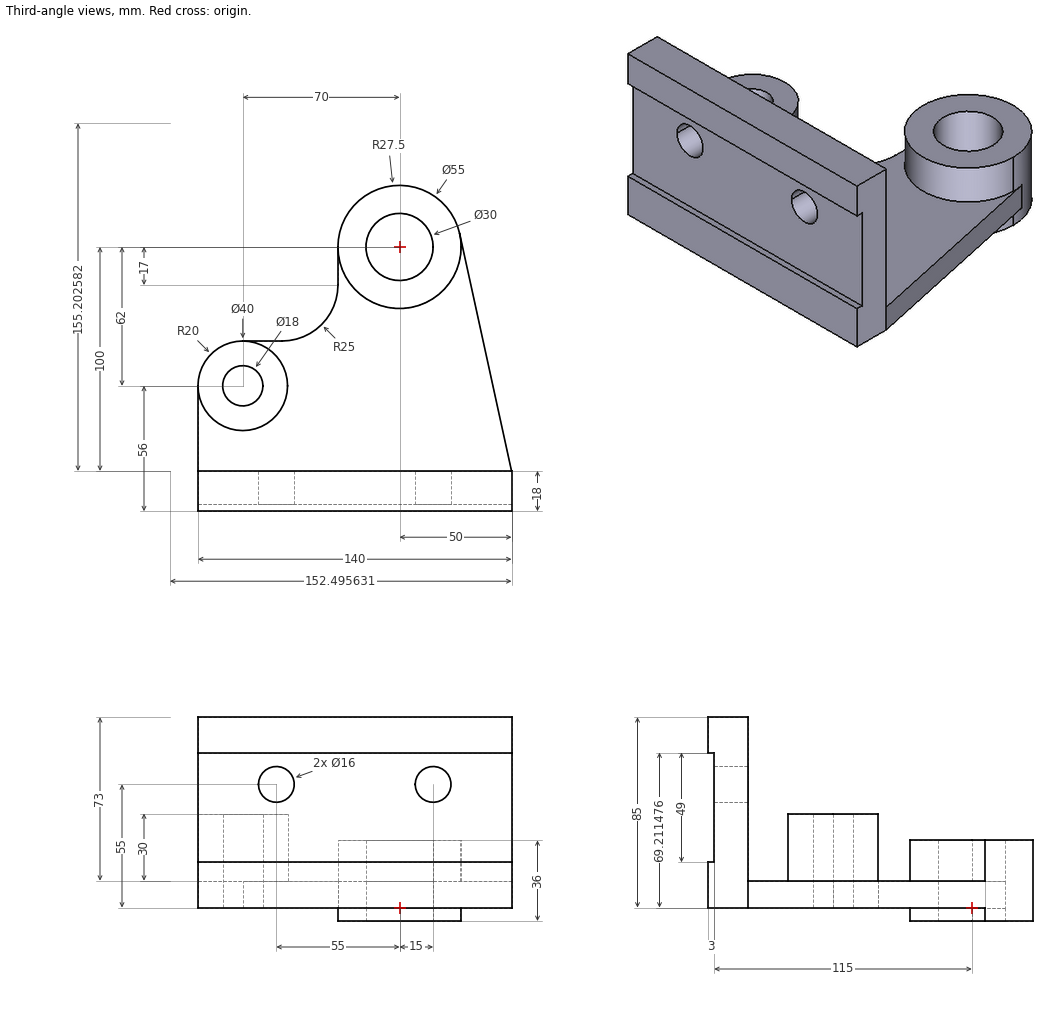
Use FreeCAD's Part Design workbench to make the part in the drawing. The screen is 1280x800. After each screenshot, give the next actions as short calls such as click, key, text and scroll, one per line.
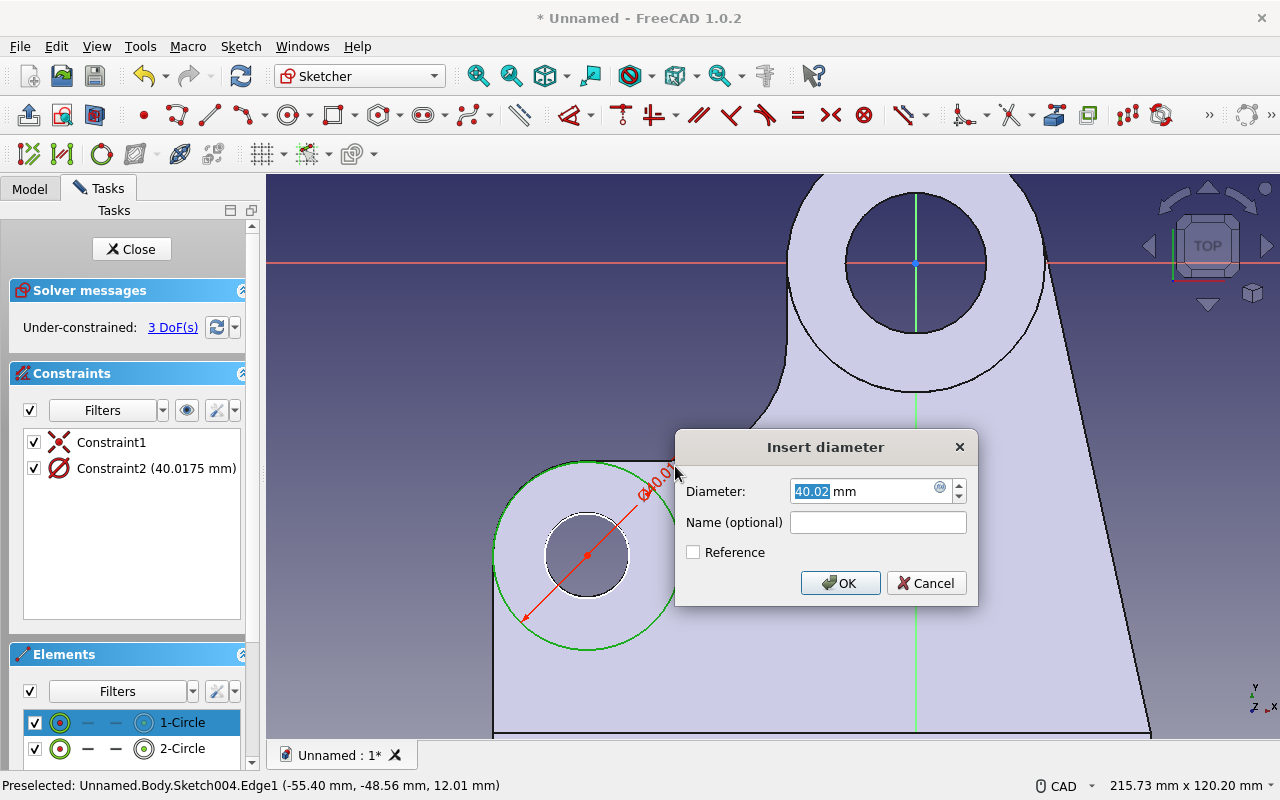
text(40)
key(Return)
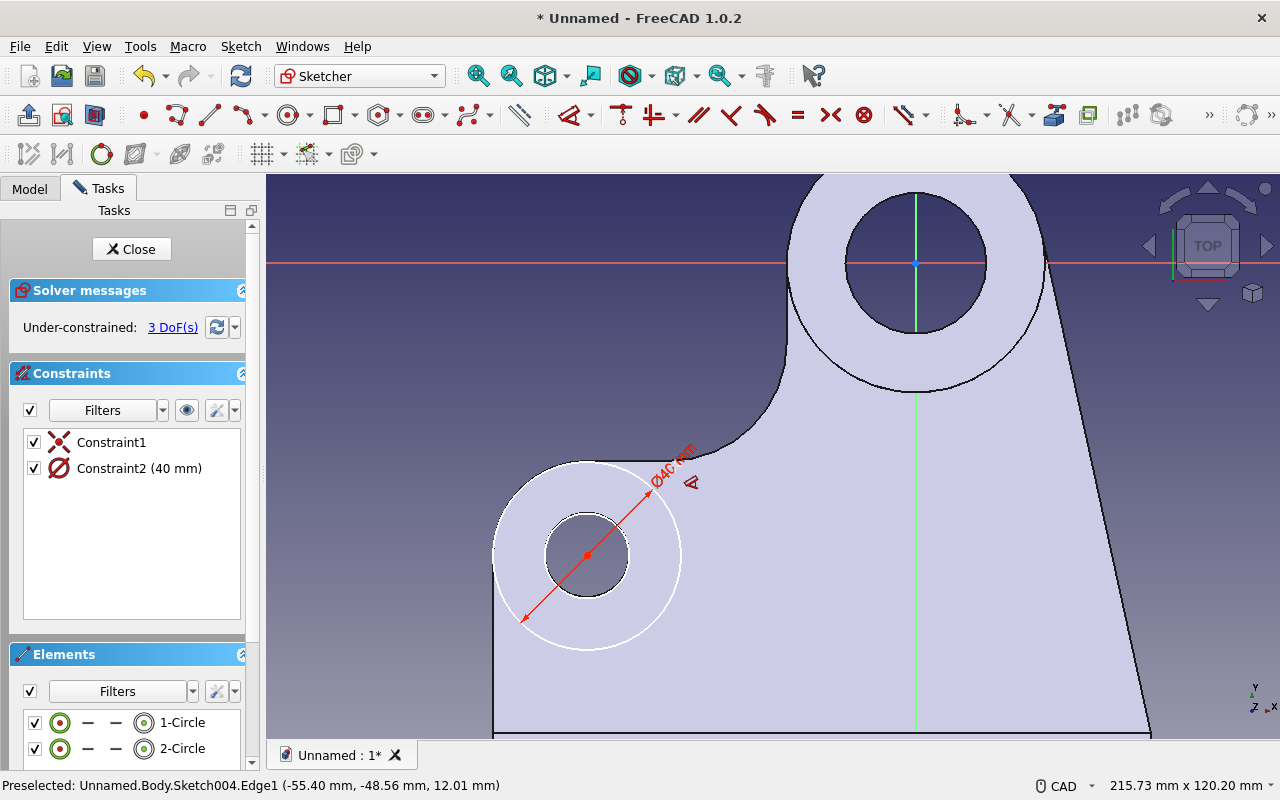
click(617, 526)
click(640, 503)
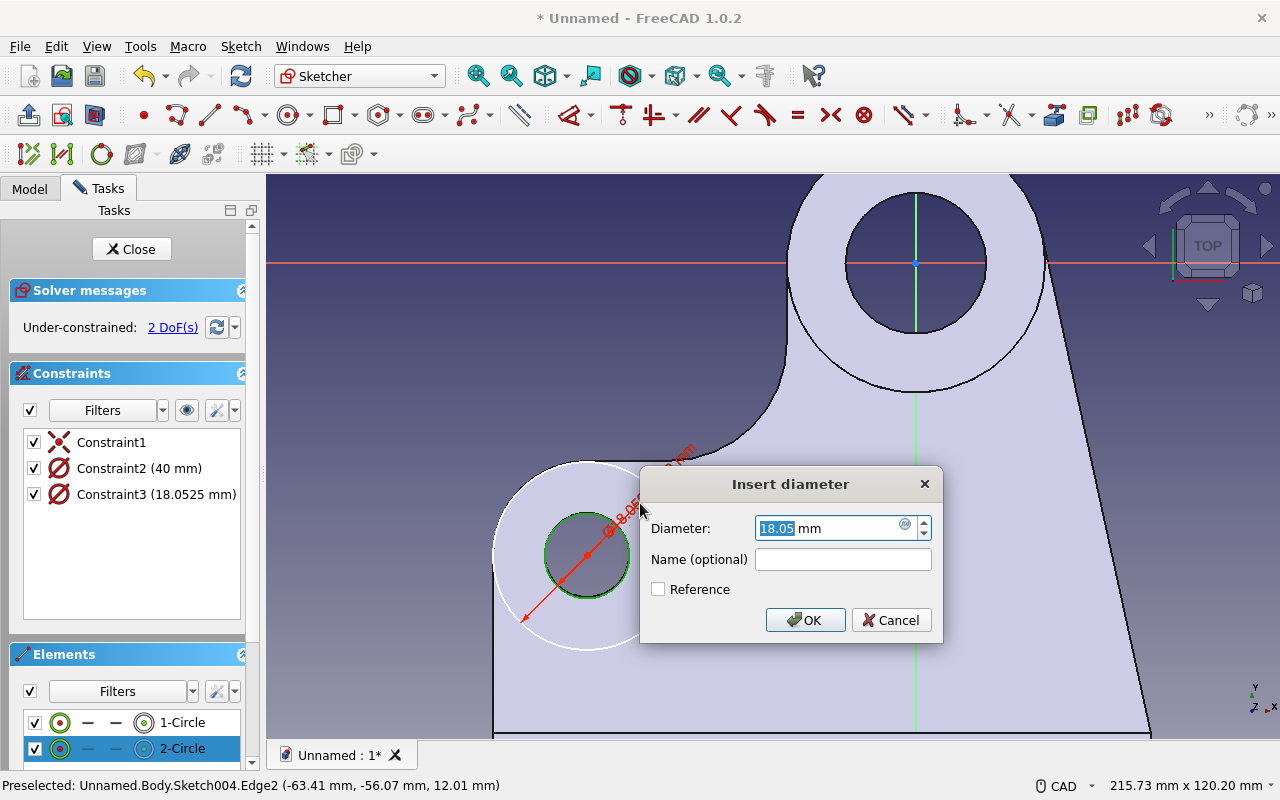
text(18)
key(Return)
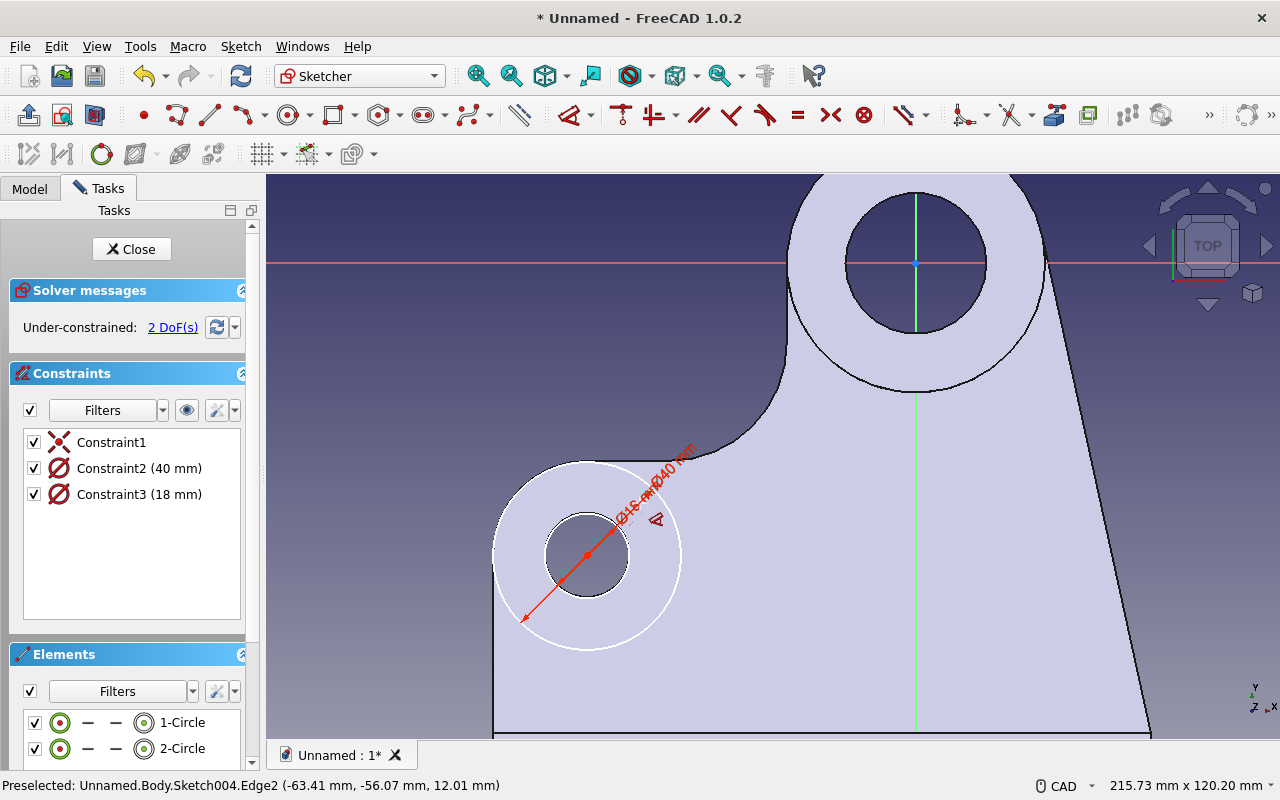
click(587, 556)
click(751, 229)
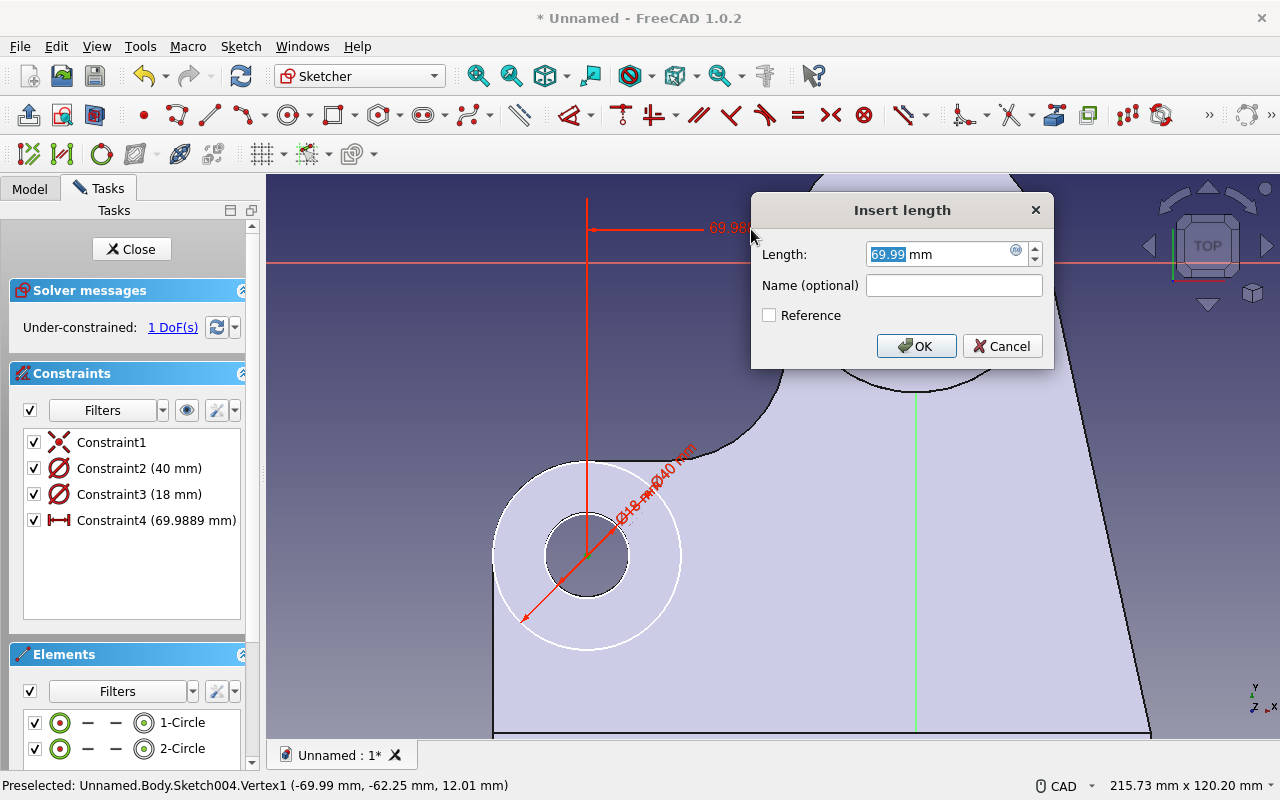
text(70)
key(Return)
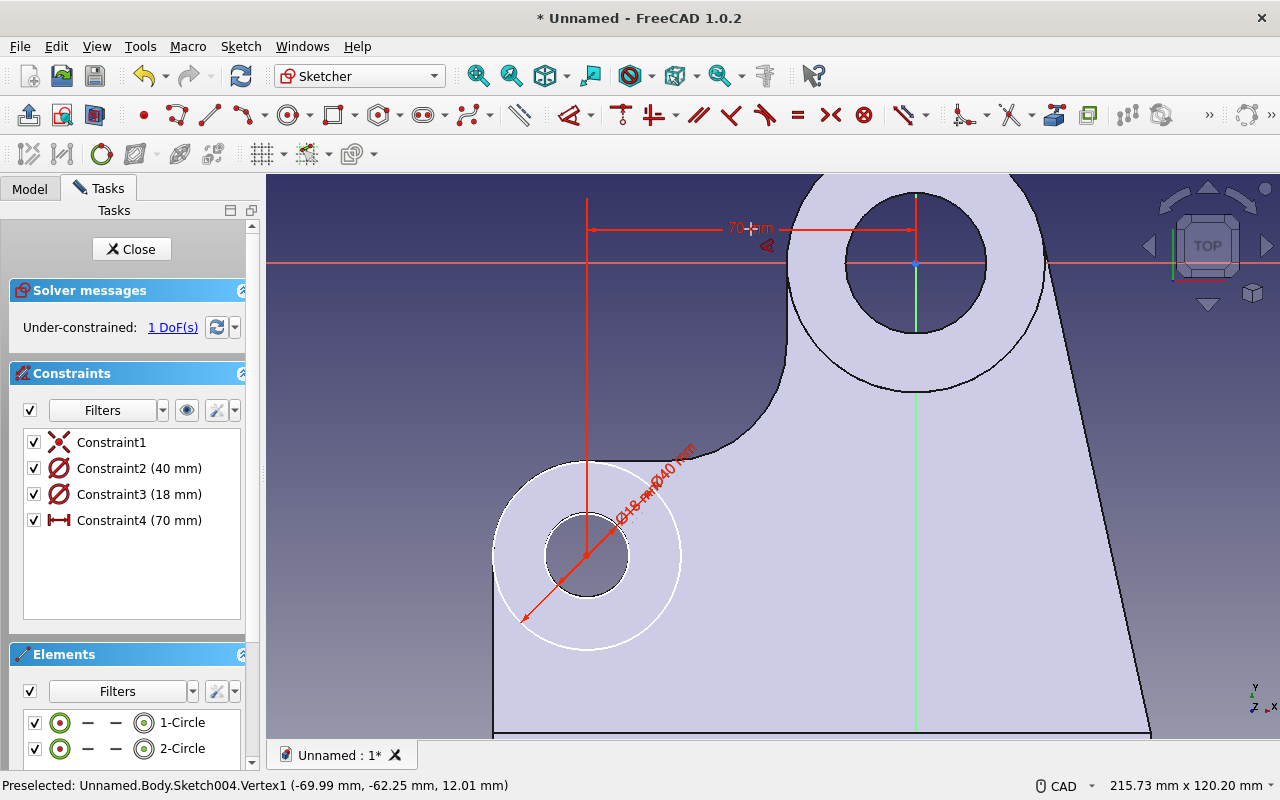
click(587, 556)
click(950, 410)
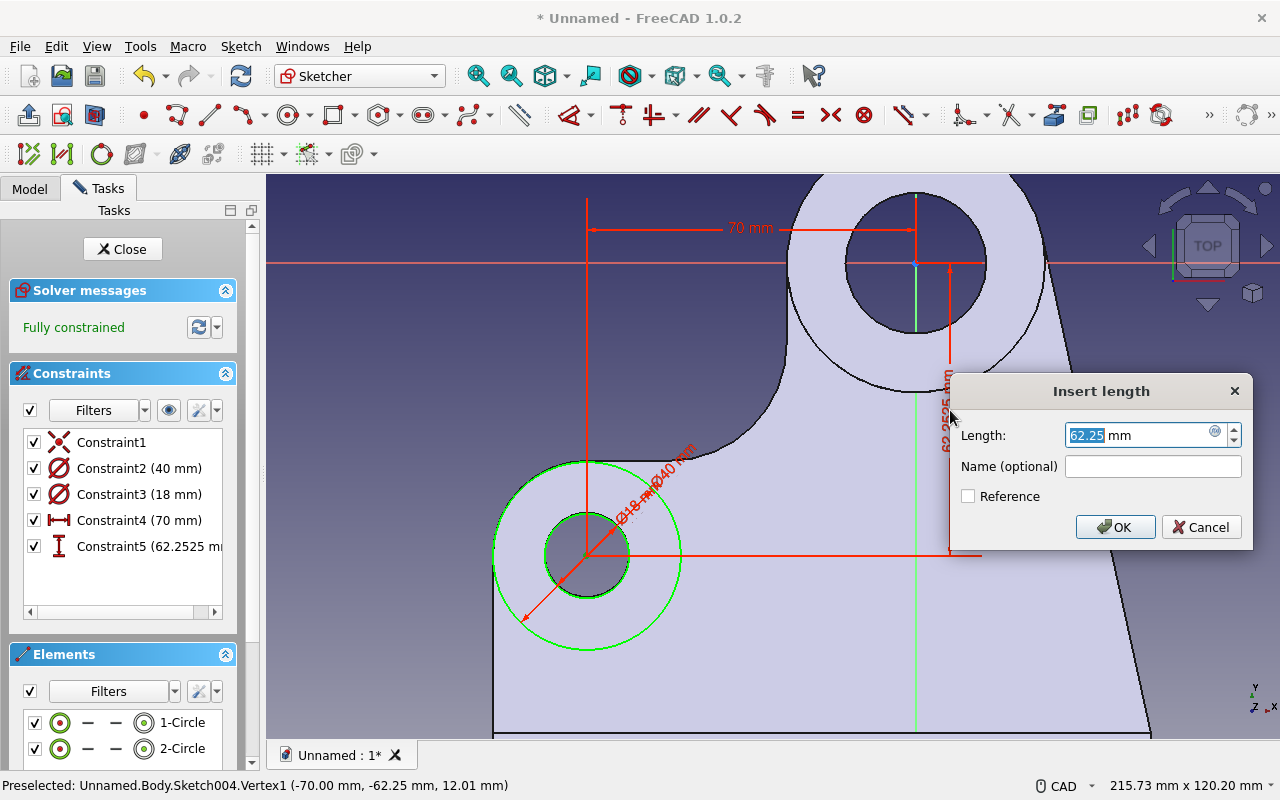
text(62)
key(Return)
key(Escape)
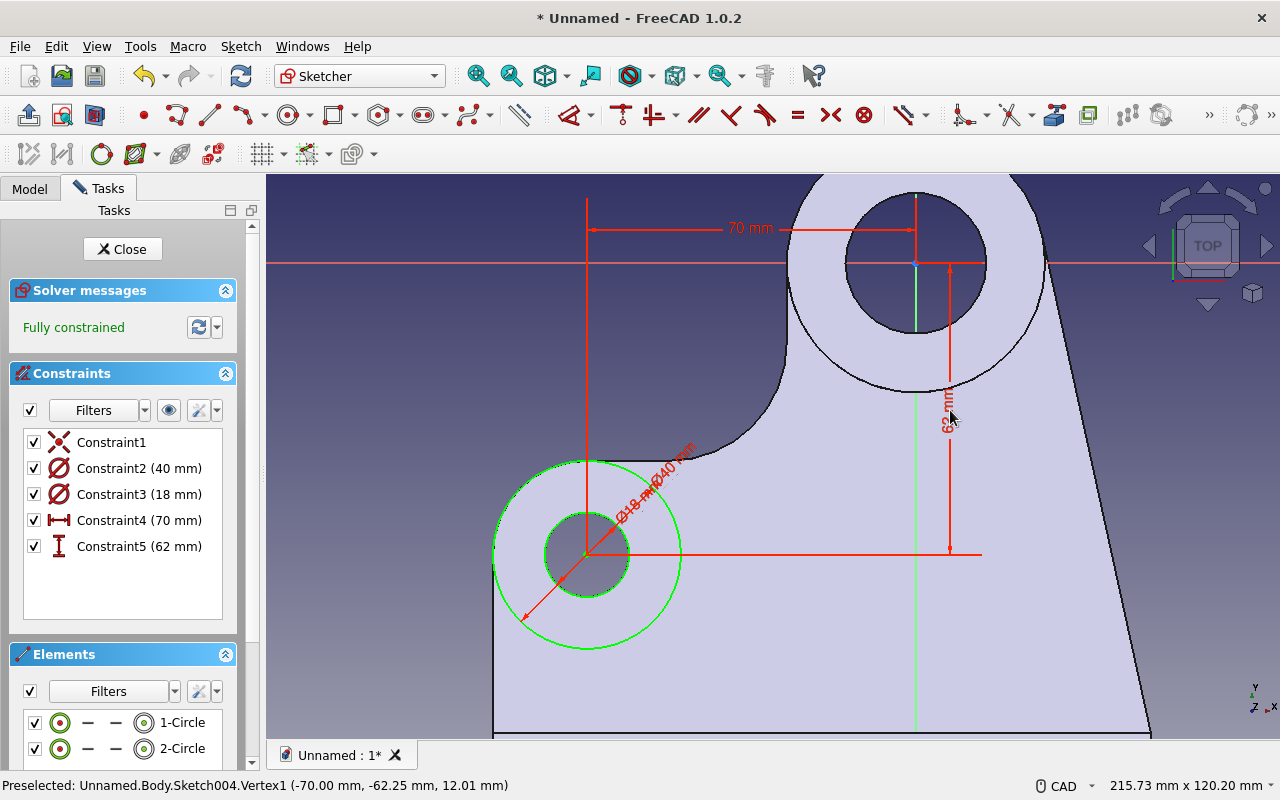
click(123, 249)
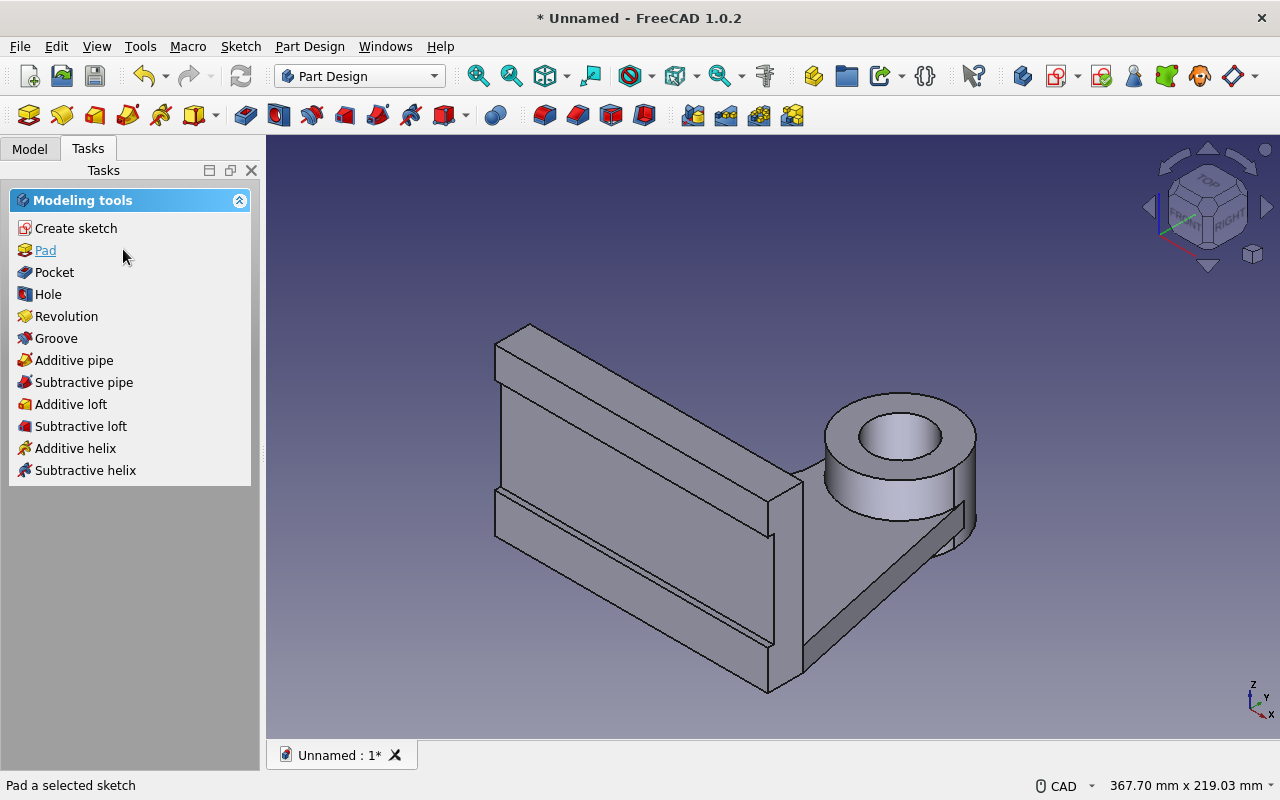
click(29, 116)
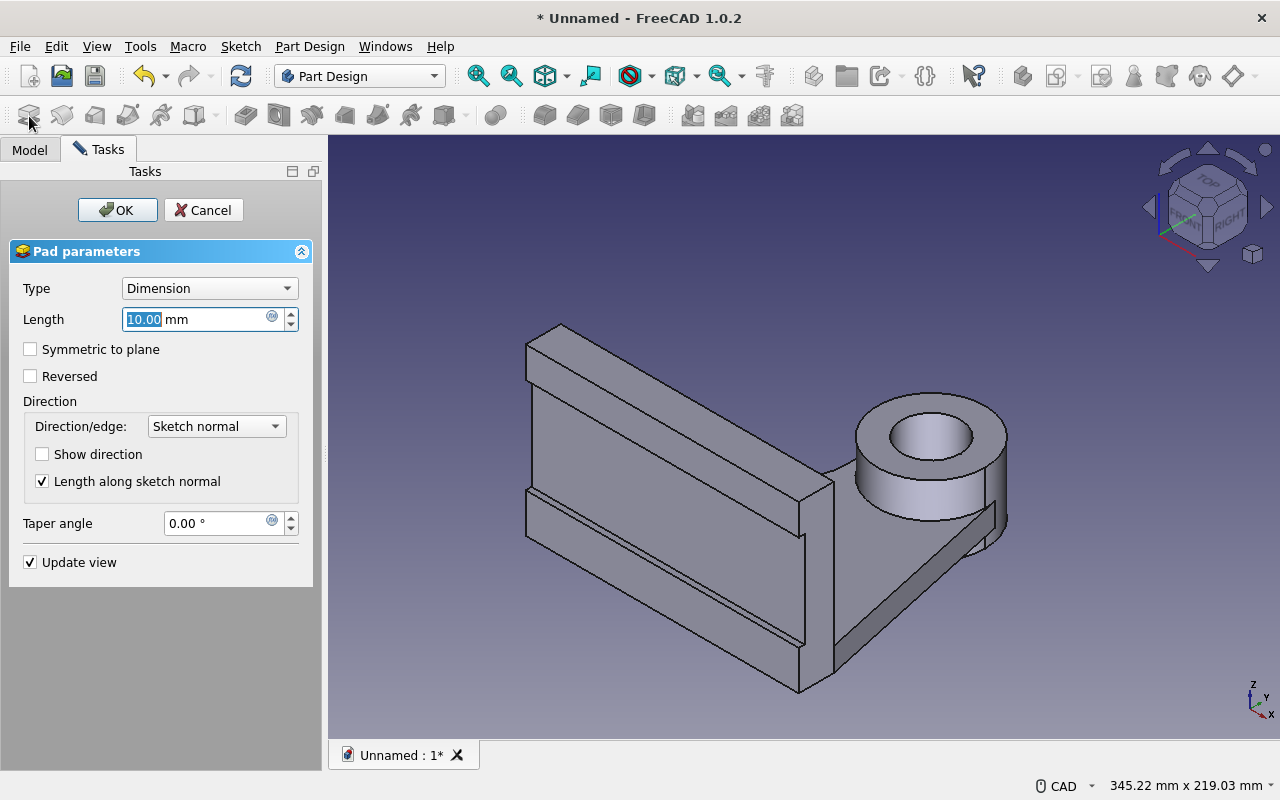
text(30)
key(Tab)